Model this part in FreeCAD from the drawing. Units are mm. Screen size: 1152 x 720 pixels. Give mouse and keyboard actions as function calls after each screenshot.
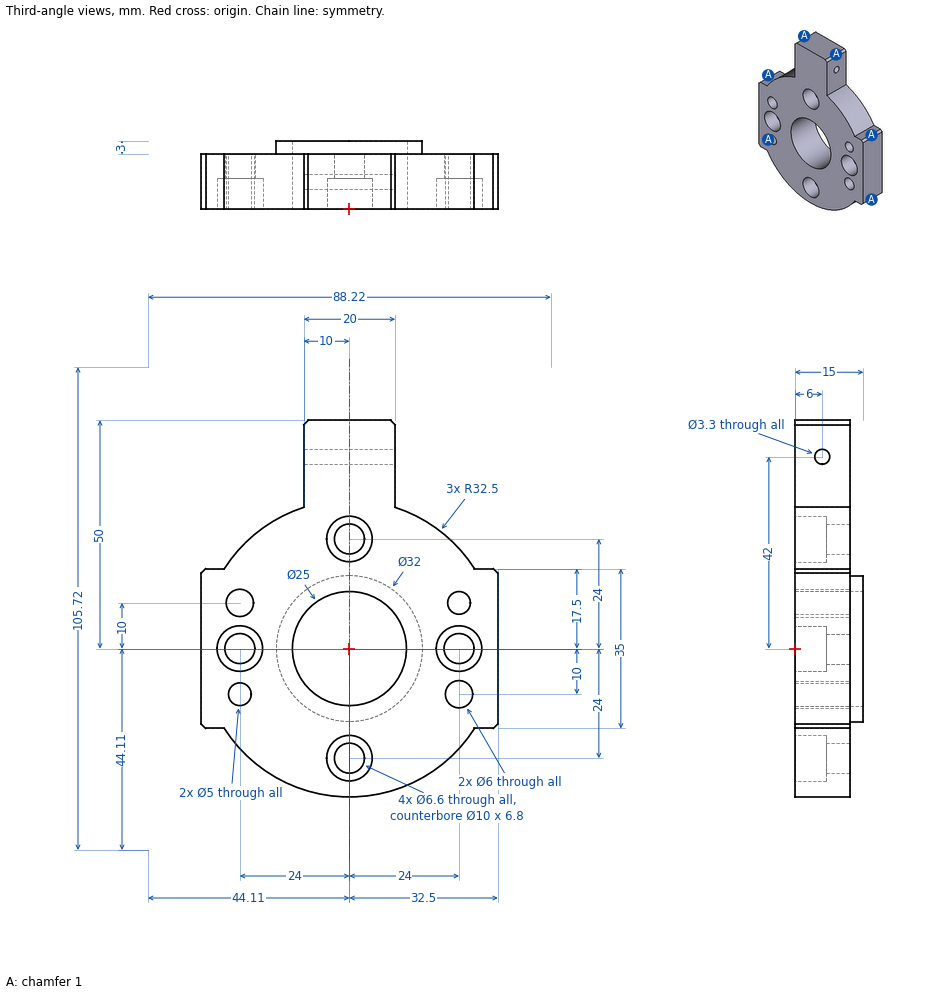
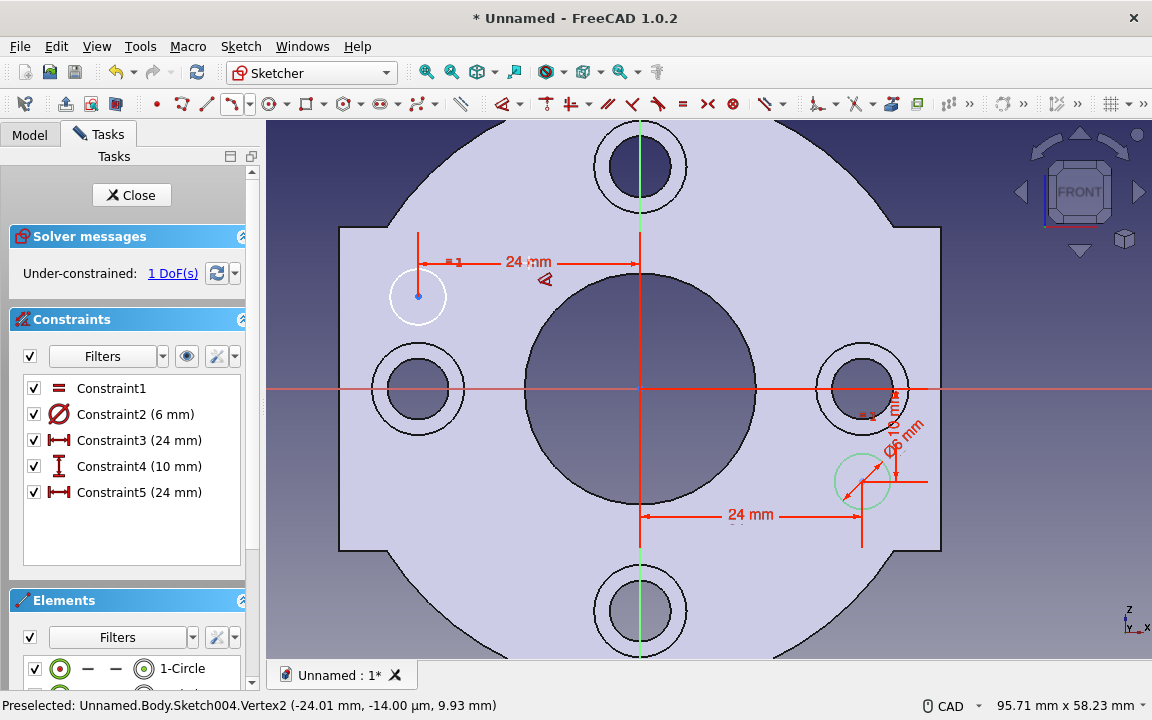
click(418, 297)
click(384, 343)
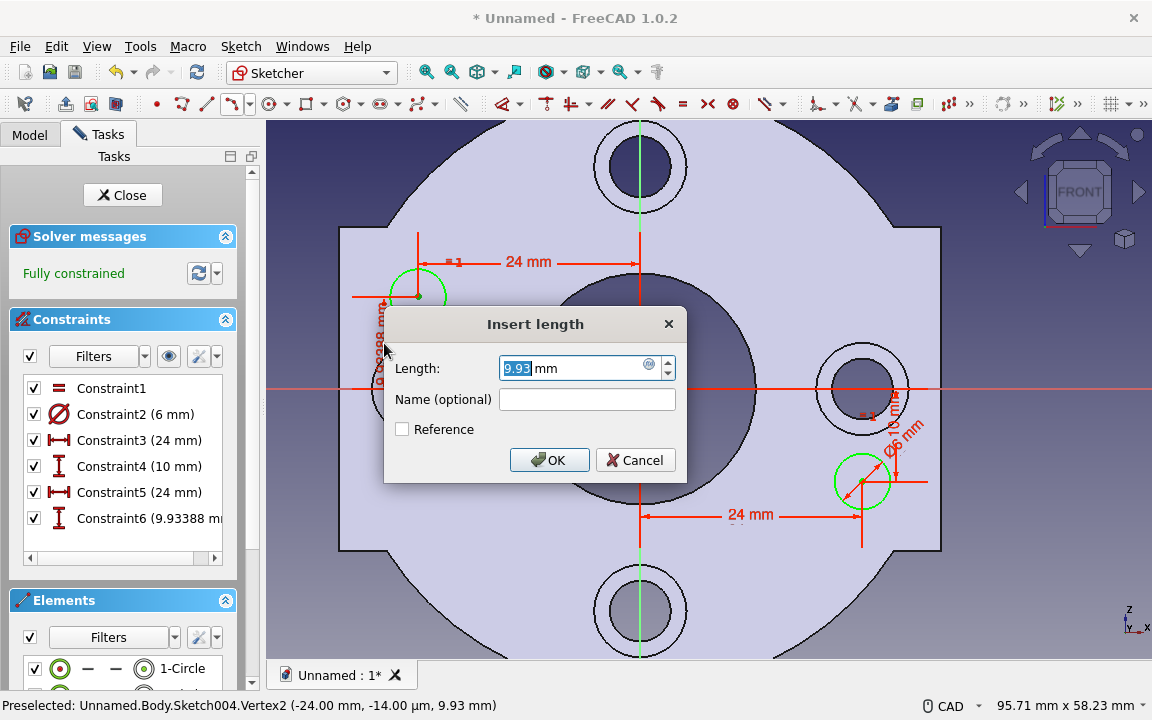
text(10)
key(Return)
key(Escape)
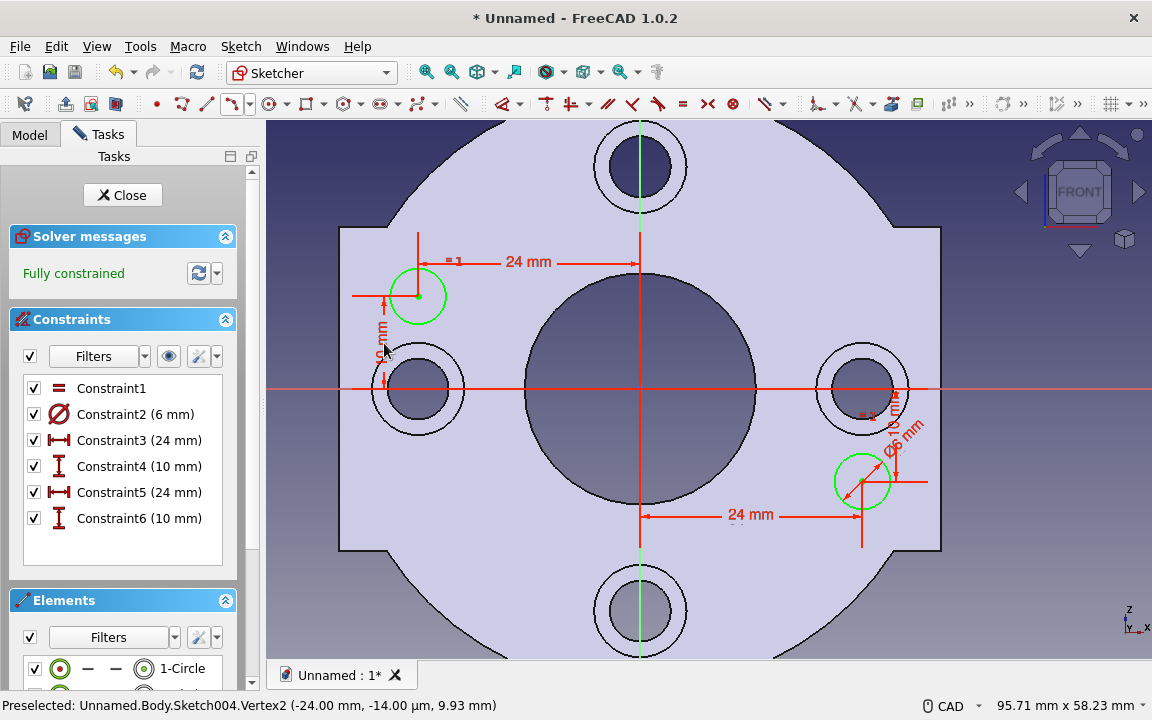
click(123, 195)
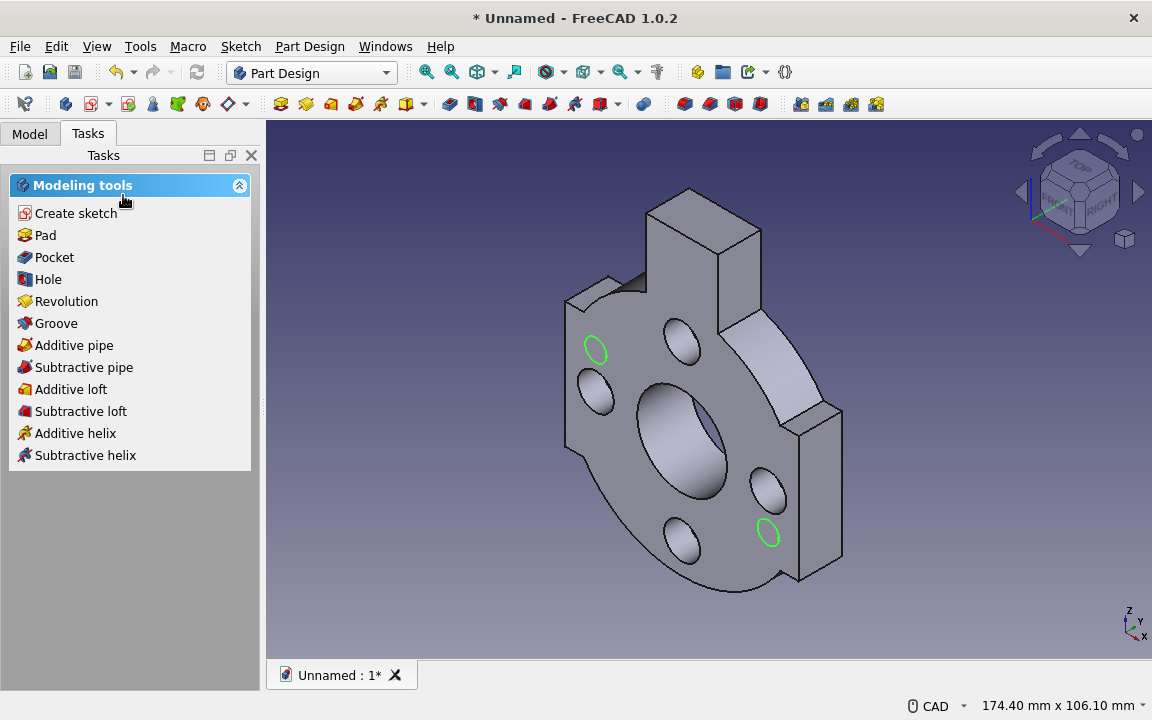
click(475, 104)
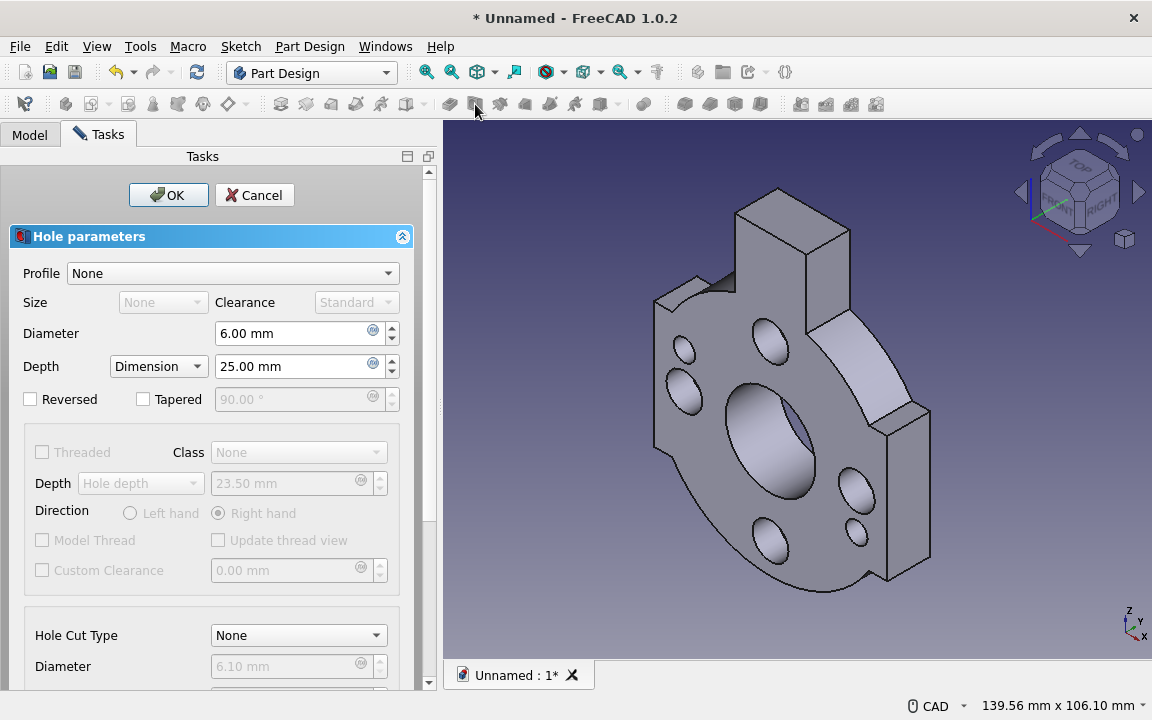
triple_click(300, 334)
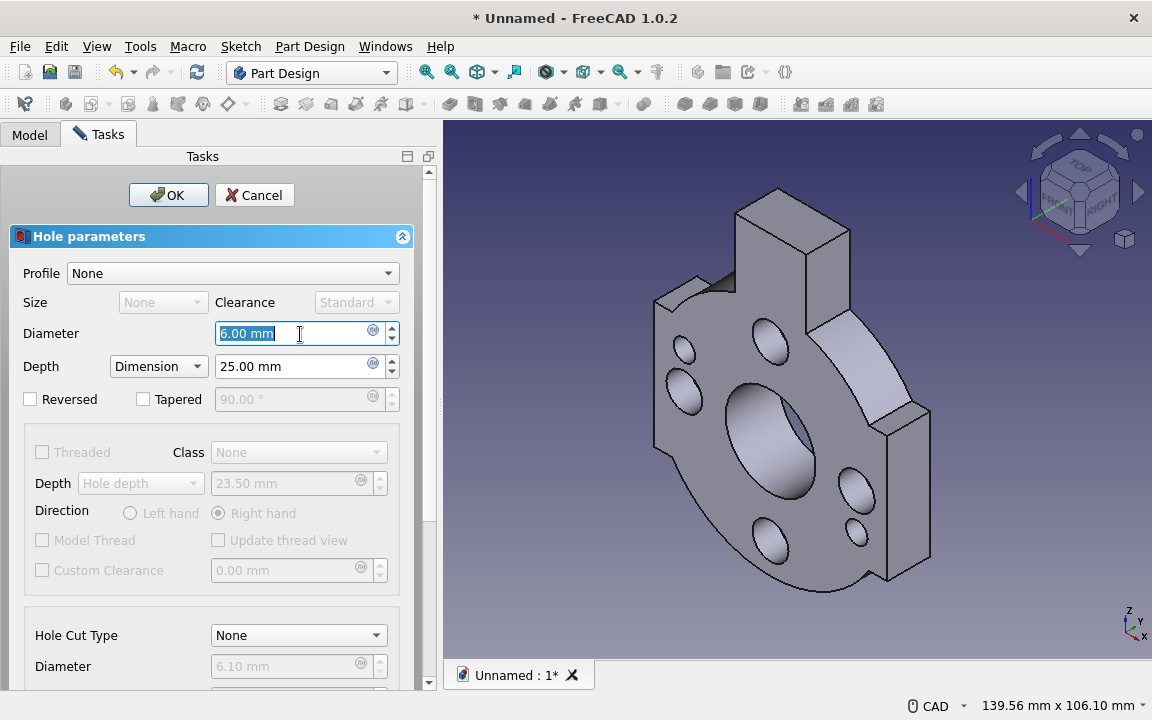
text(6)
key(Tab)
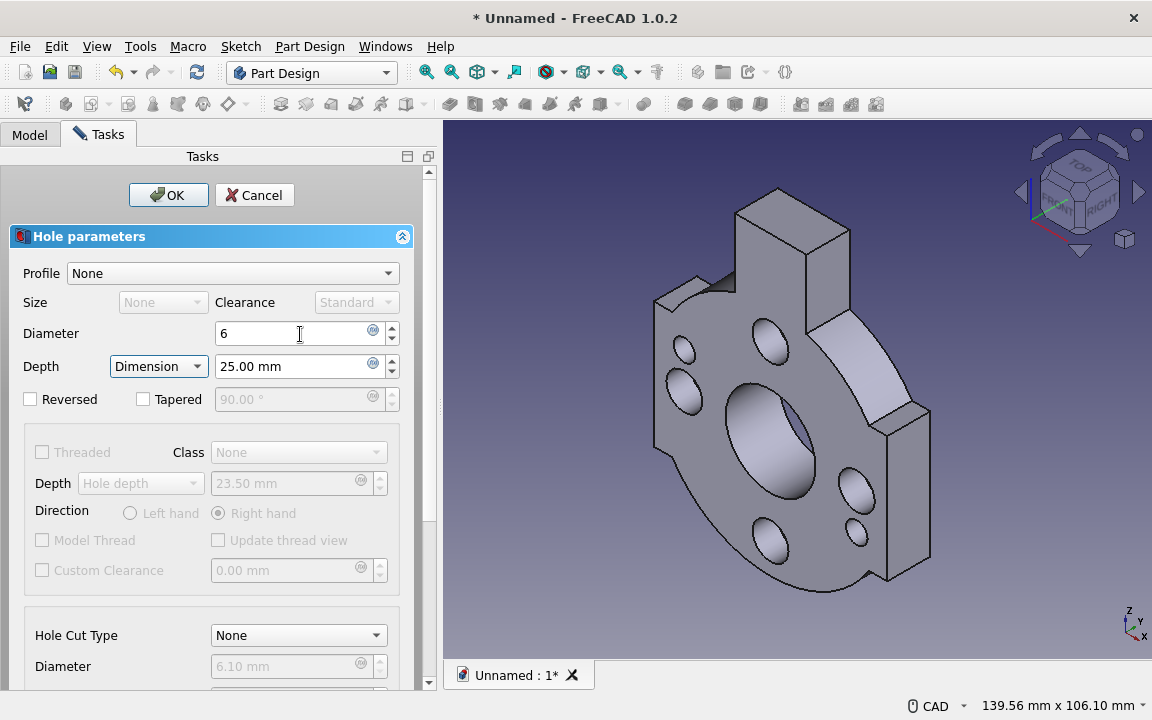
click(160, 366)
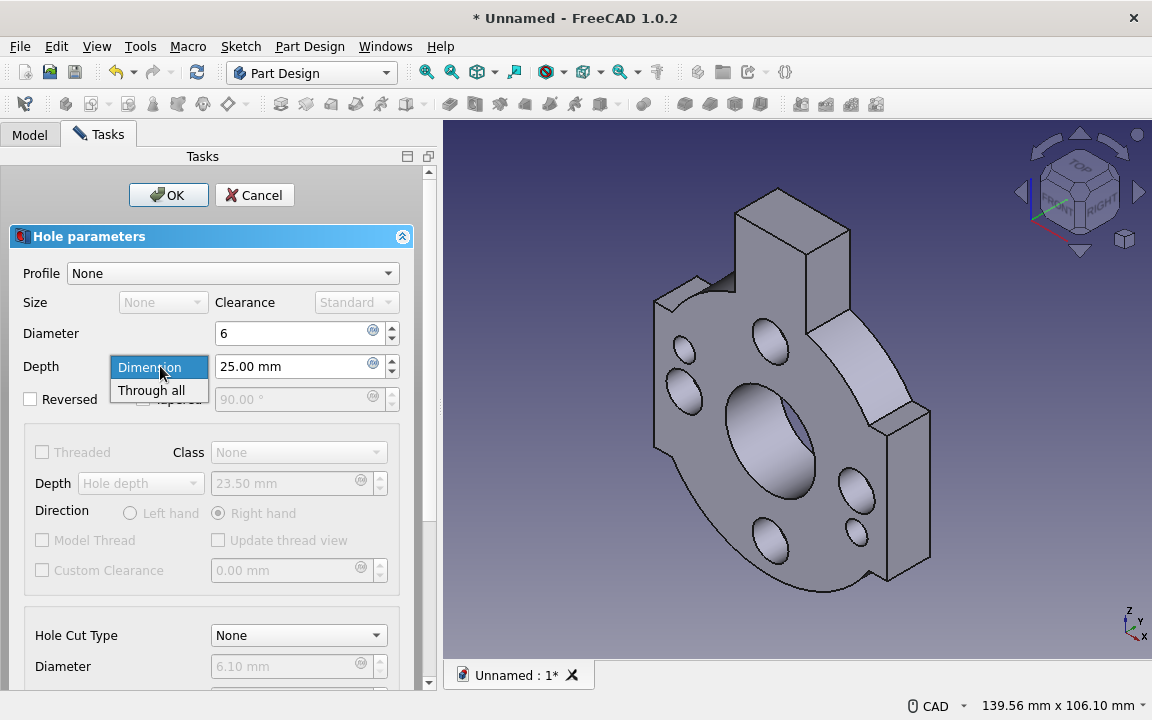
click(158, 390)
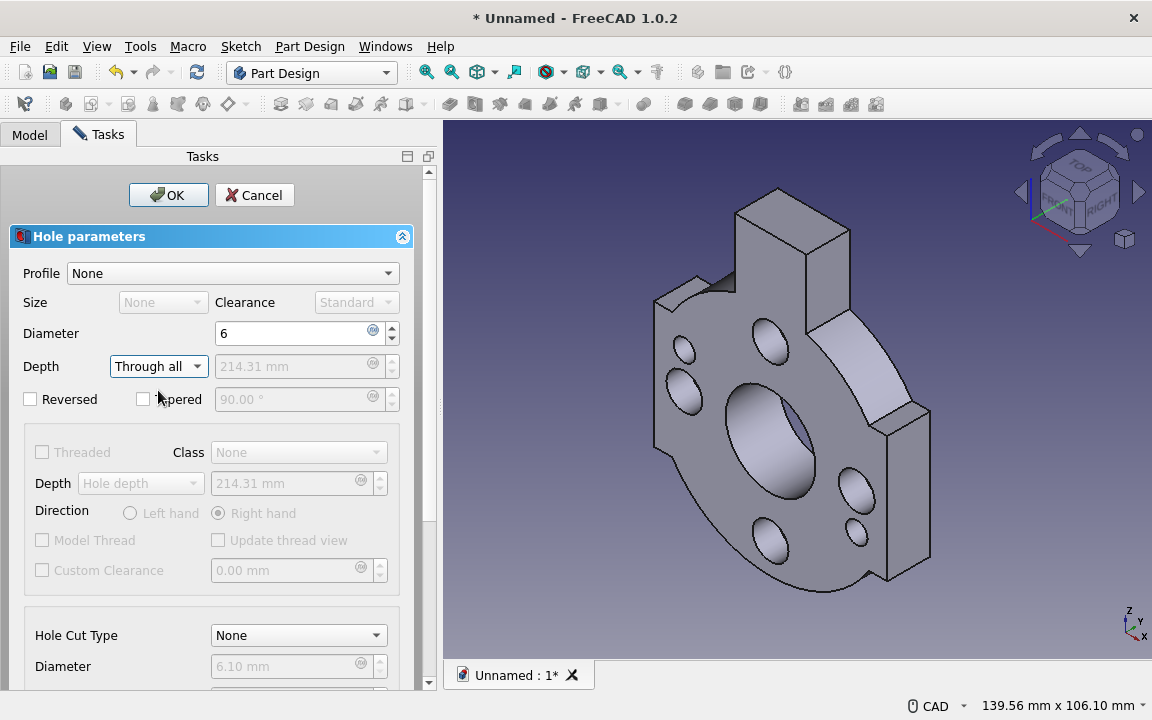
click(169, 195)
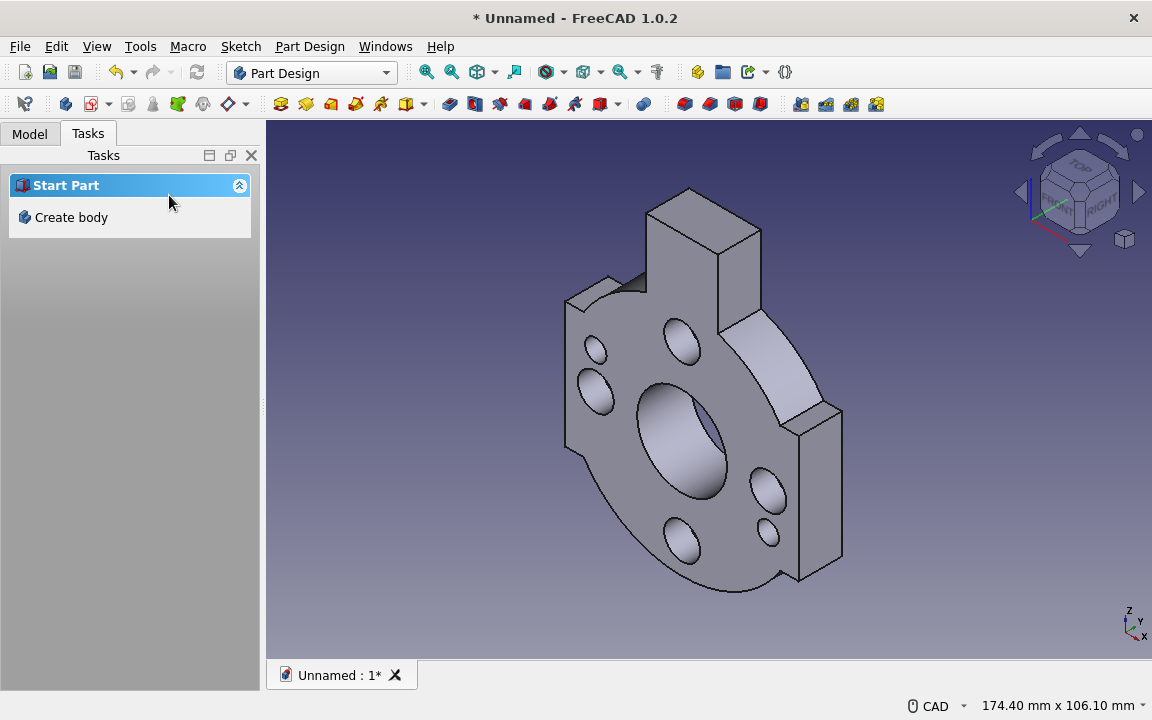
key(6)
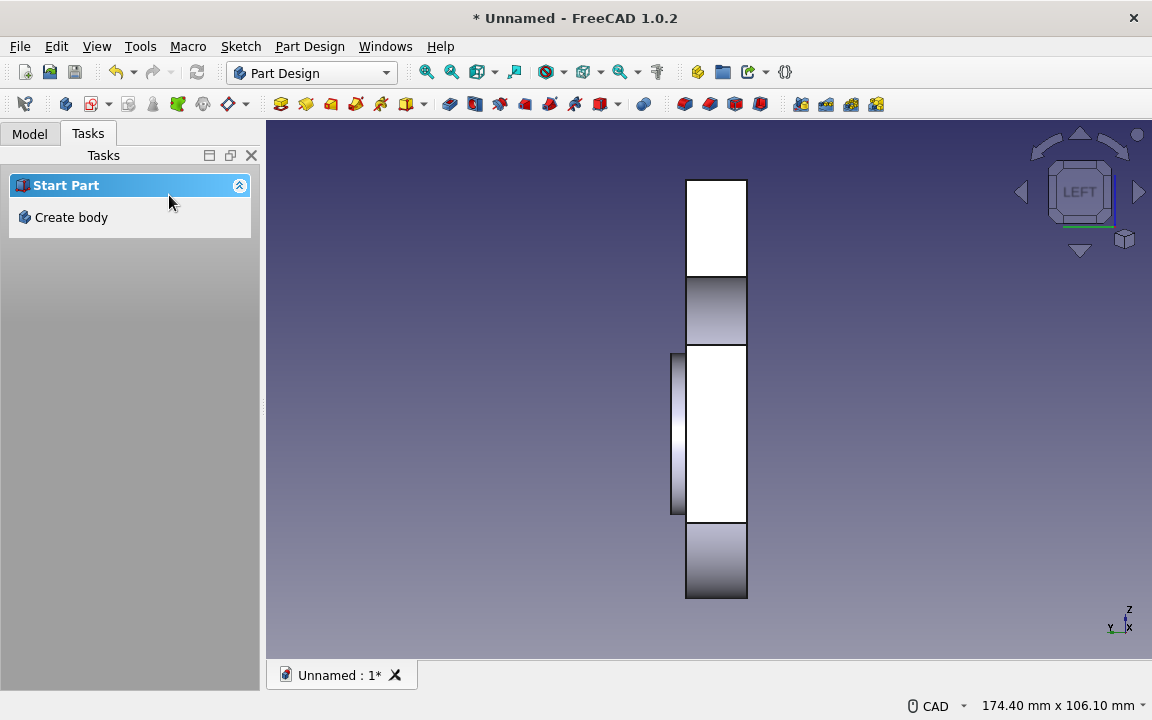
click(717, 241)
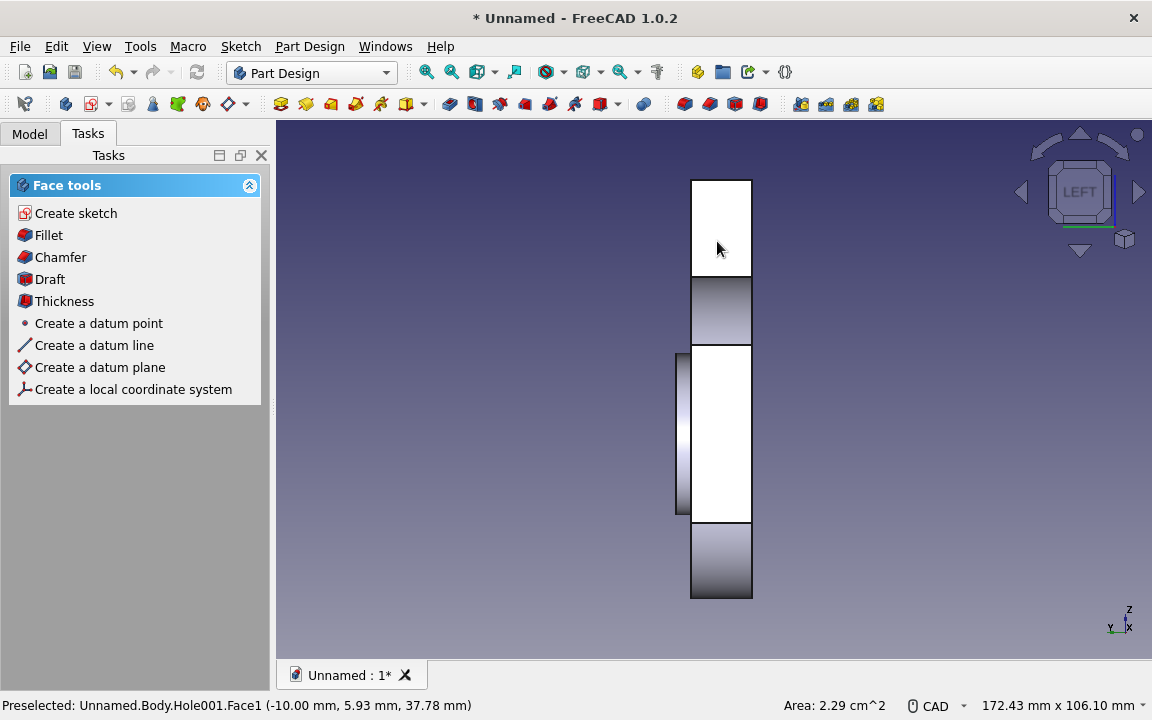
click(90, 104)